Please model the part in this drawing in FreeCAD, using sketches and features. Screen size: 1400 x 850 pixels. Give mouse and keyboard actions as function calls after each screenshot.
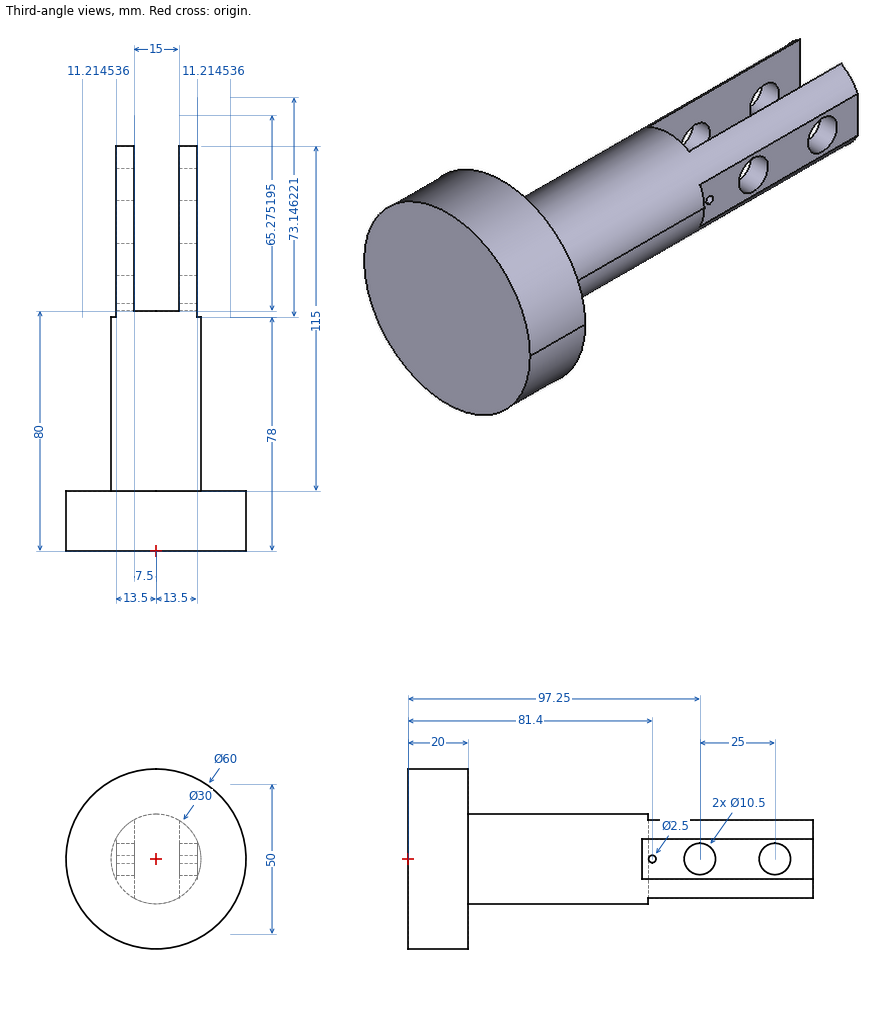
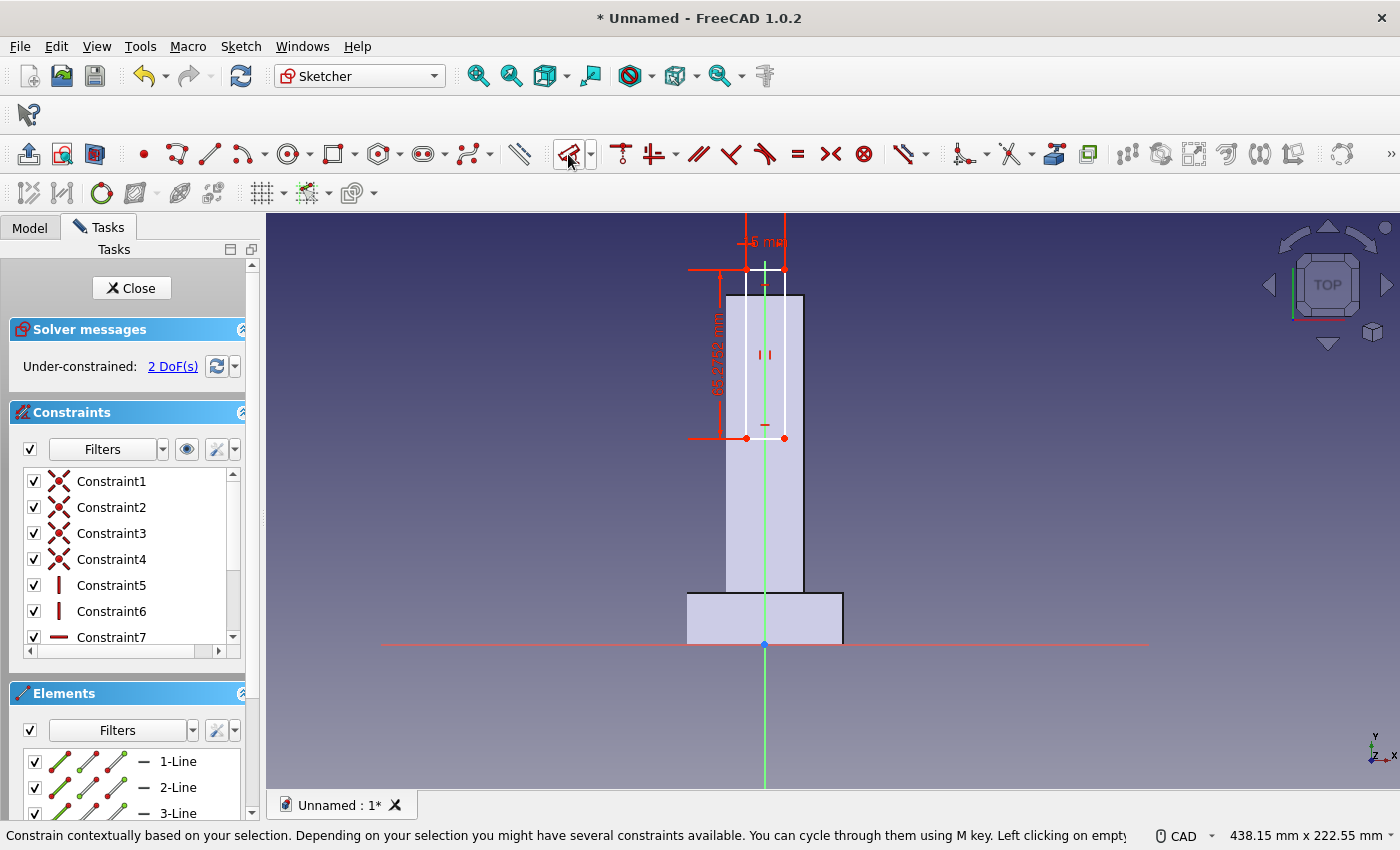
click(746, 439)
click(712, 542)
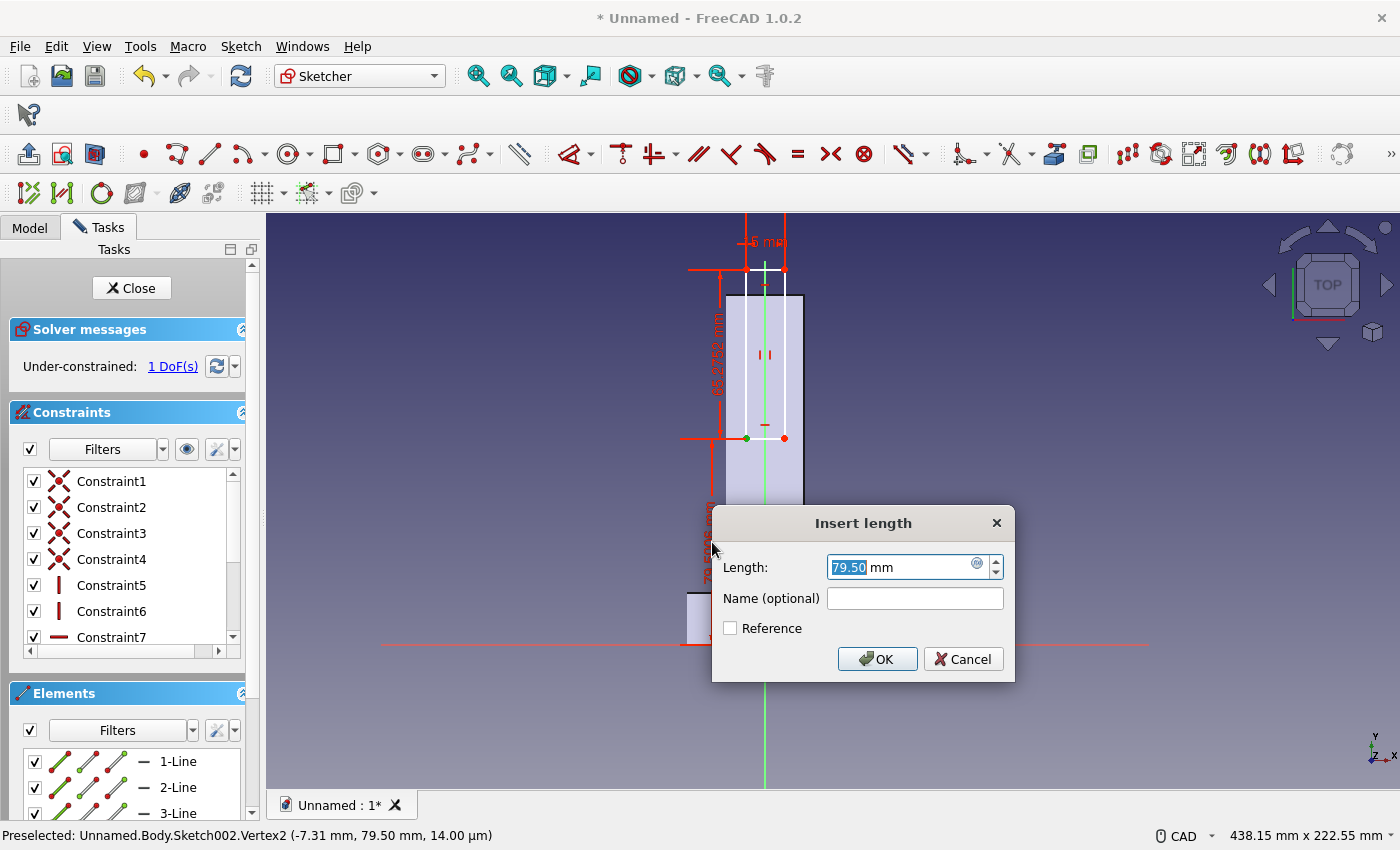
text(80)
key(Return)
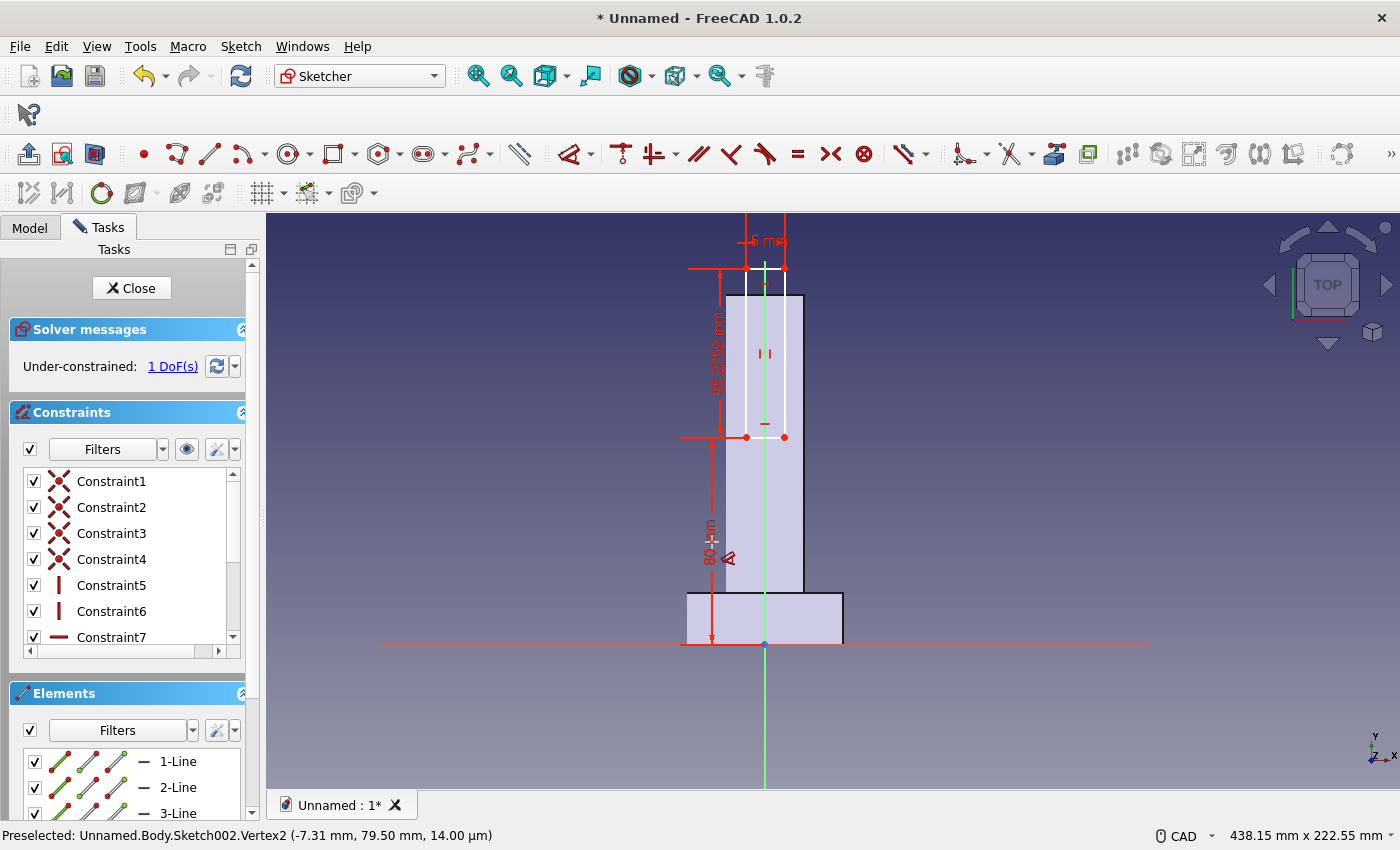
scroll(746, 269, up, 4)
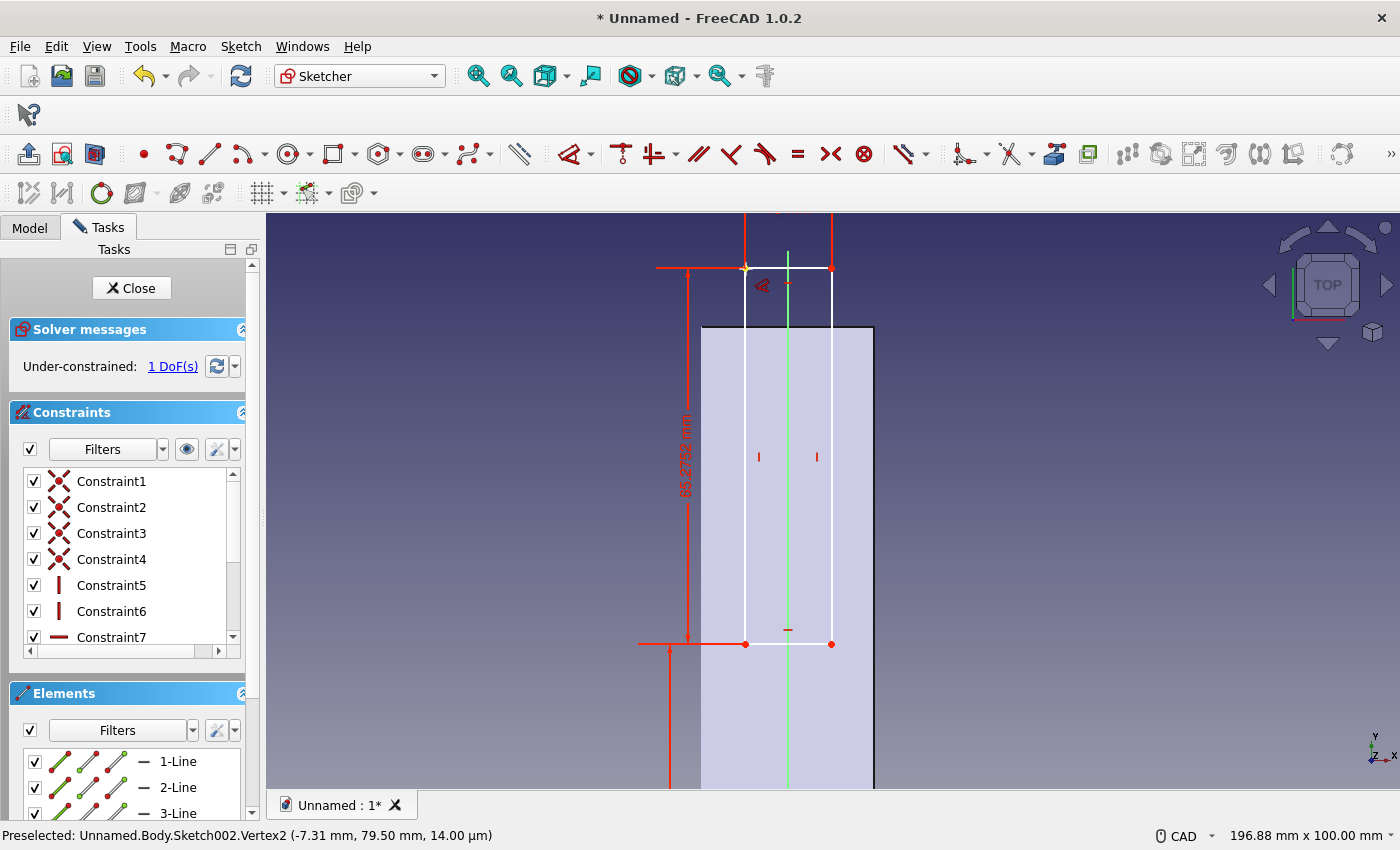
click(745, 268)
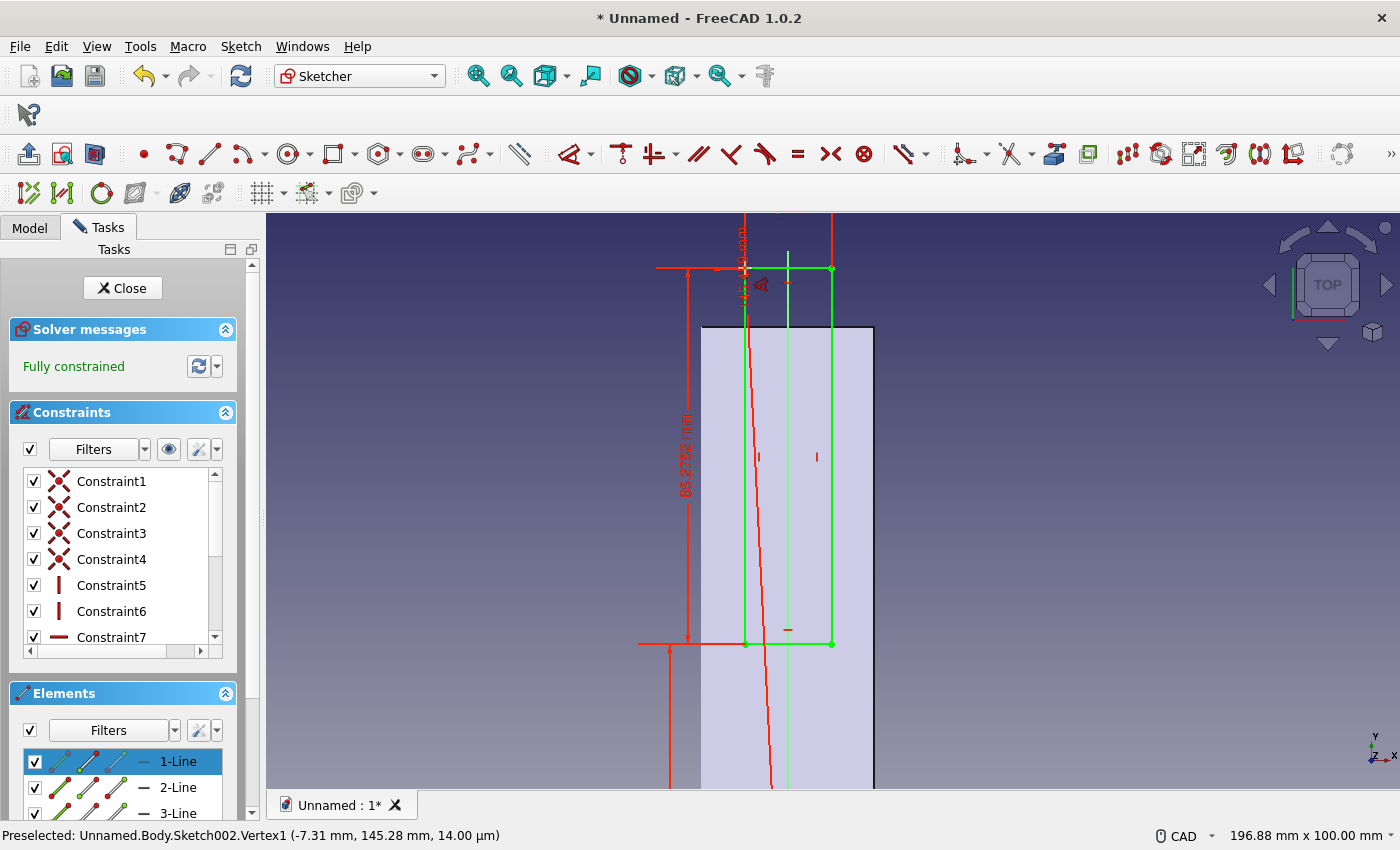
key(Escape)
key(Escape)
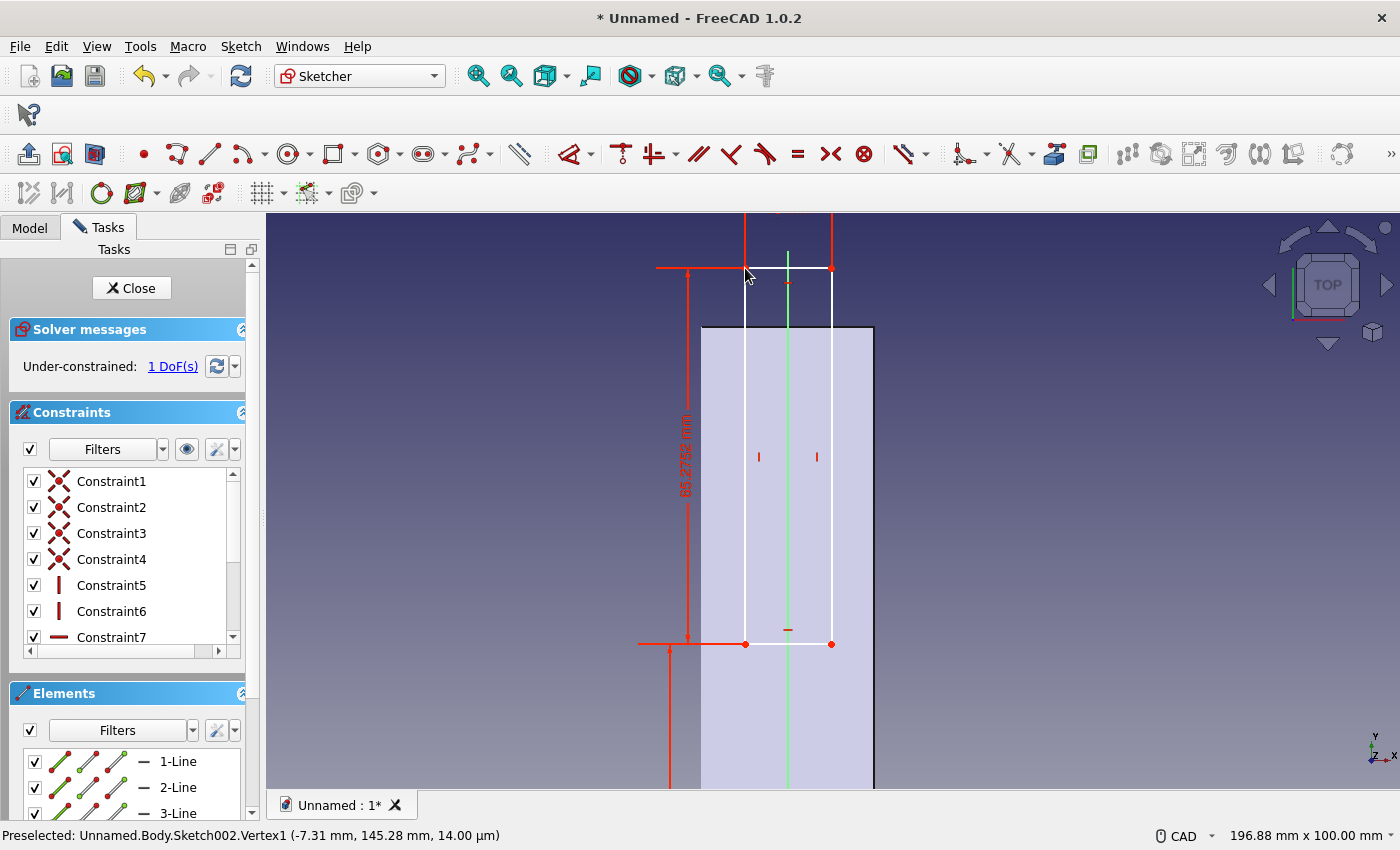
click(745, 268)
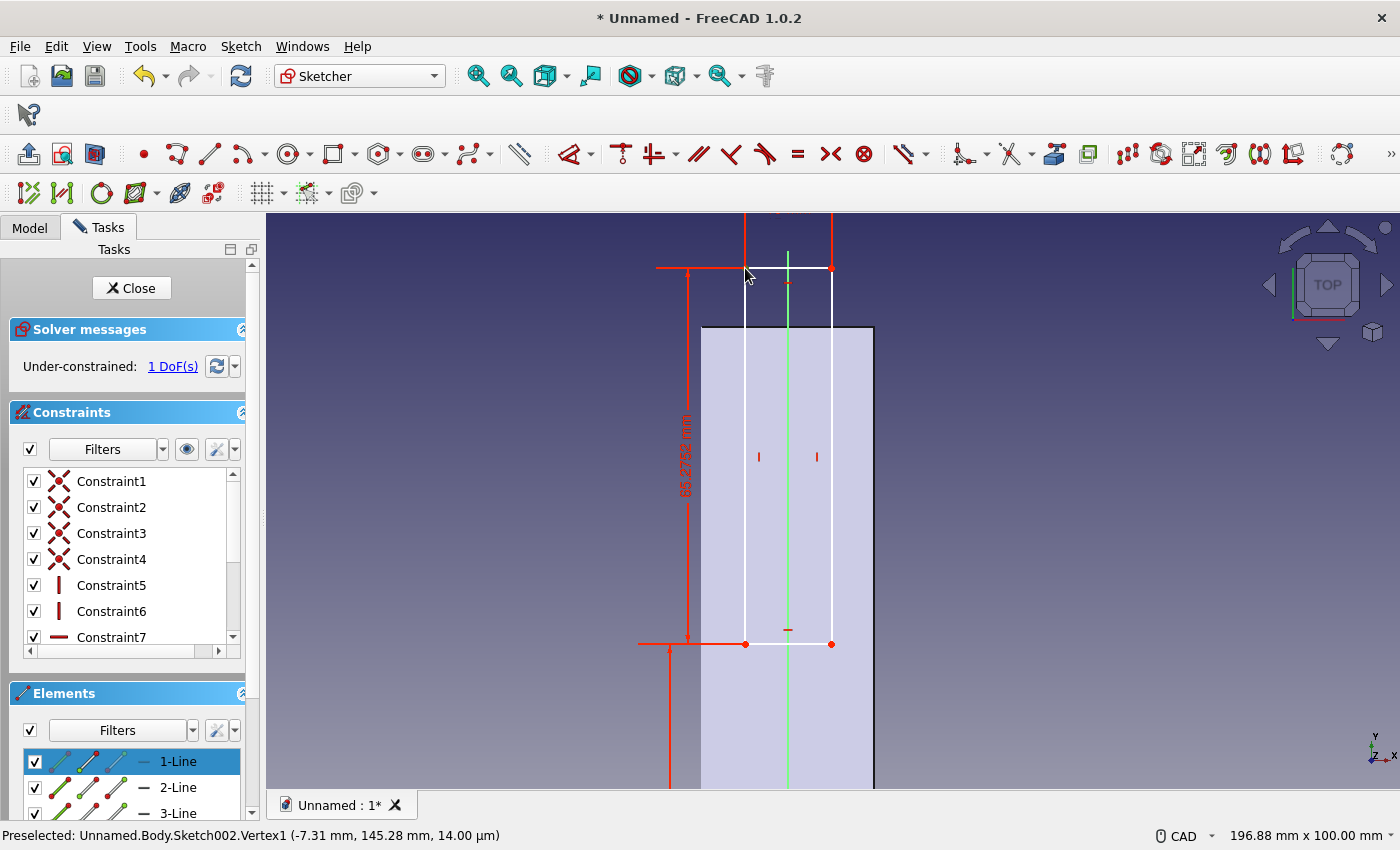
click(590, 154)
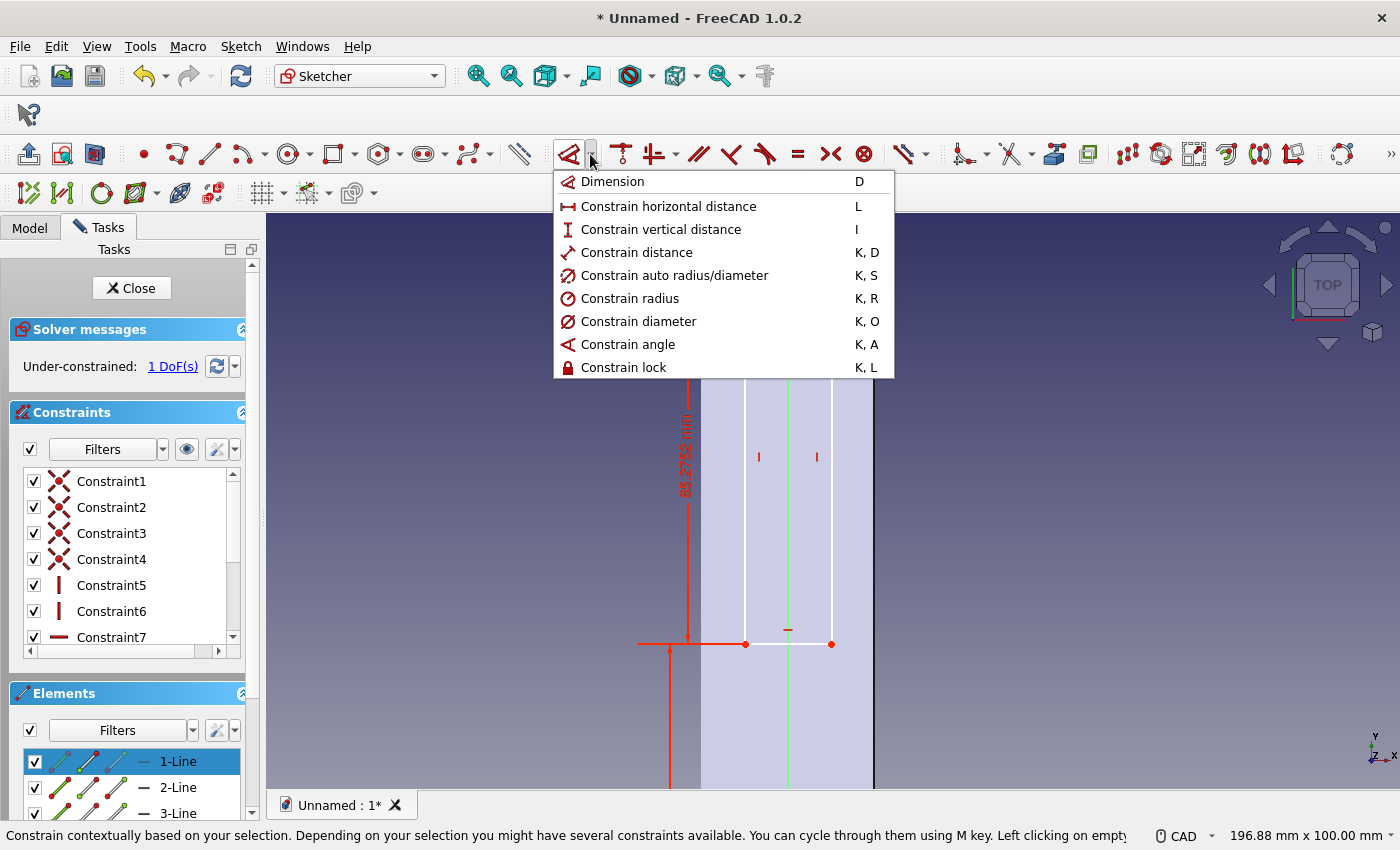
click(724, 206)